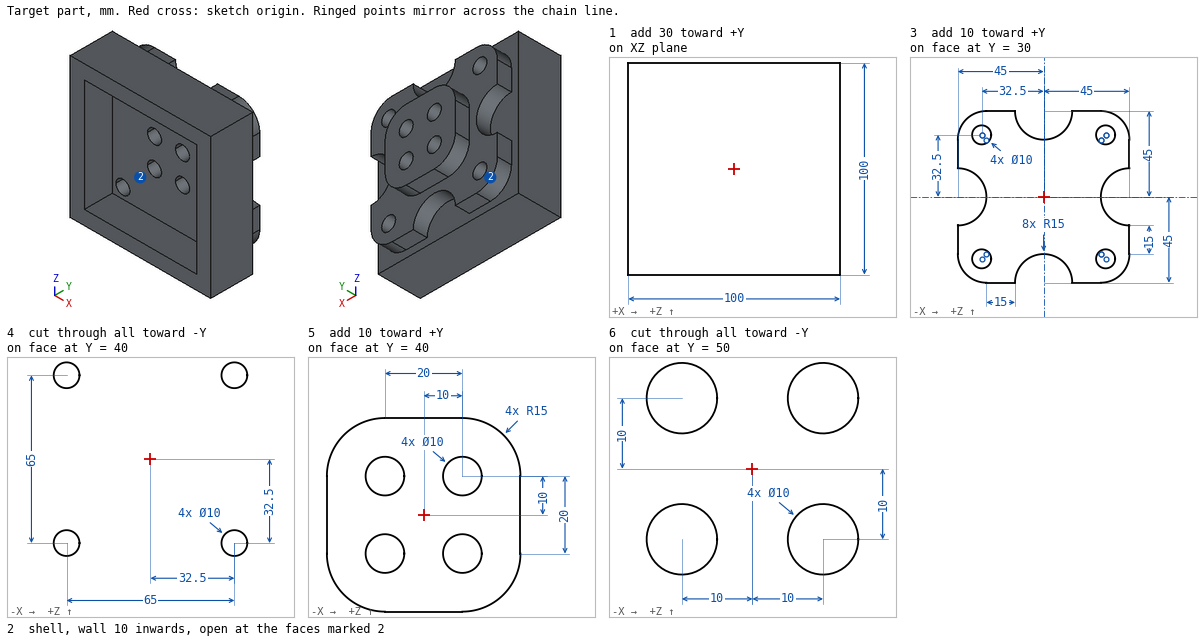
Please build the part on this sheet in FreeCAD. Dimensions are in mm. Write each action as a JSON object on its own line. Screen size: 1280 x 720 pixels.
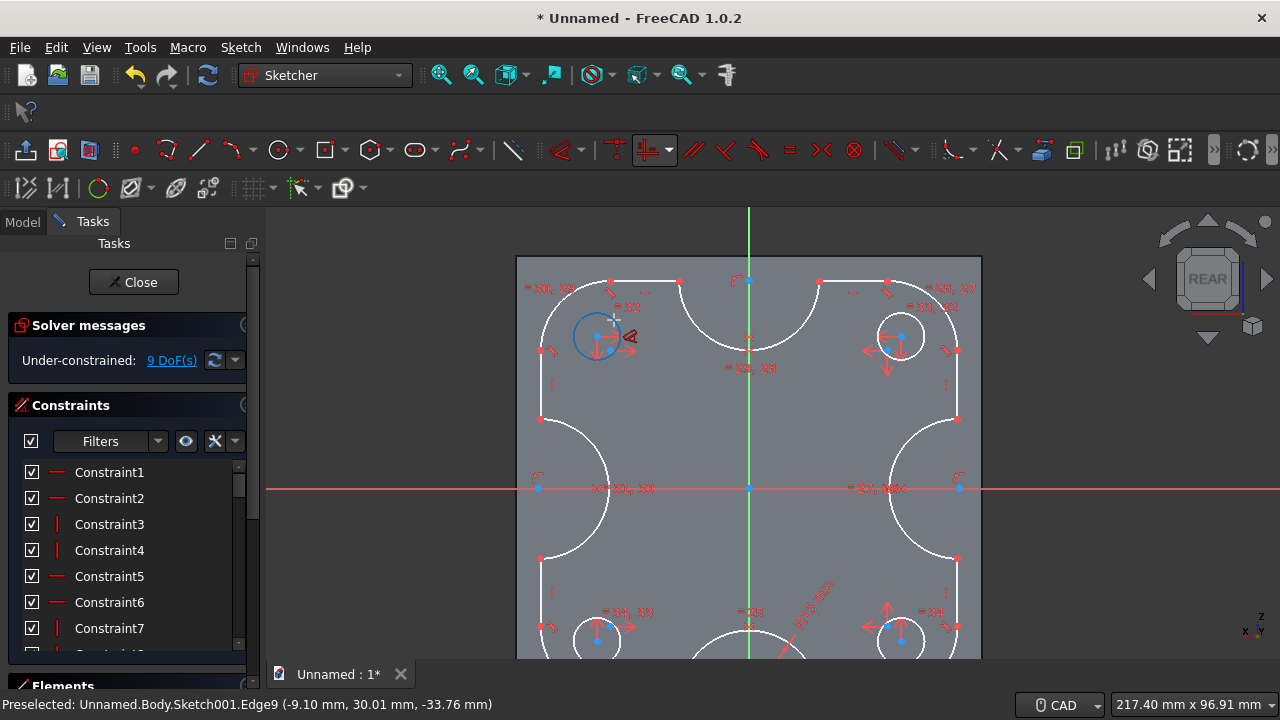
{"action": "left_click", "coordinate": [614, 320]}
{"action": "left_click", "coordinate": [637, 298]}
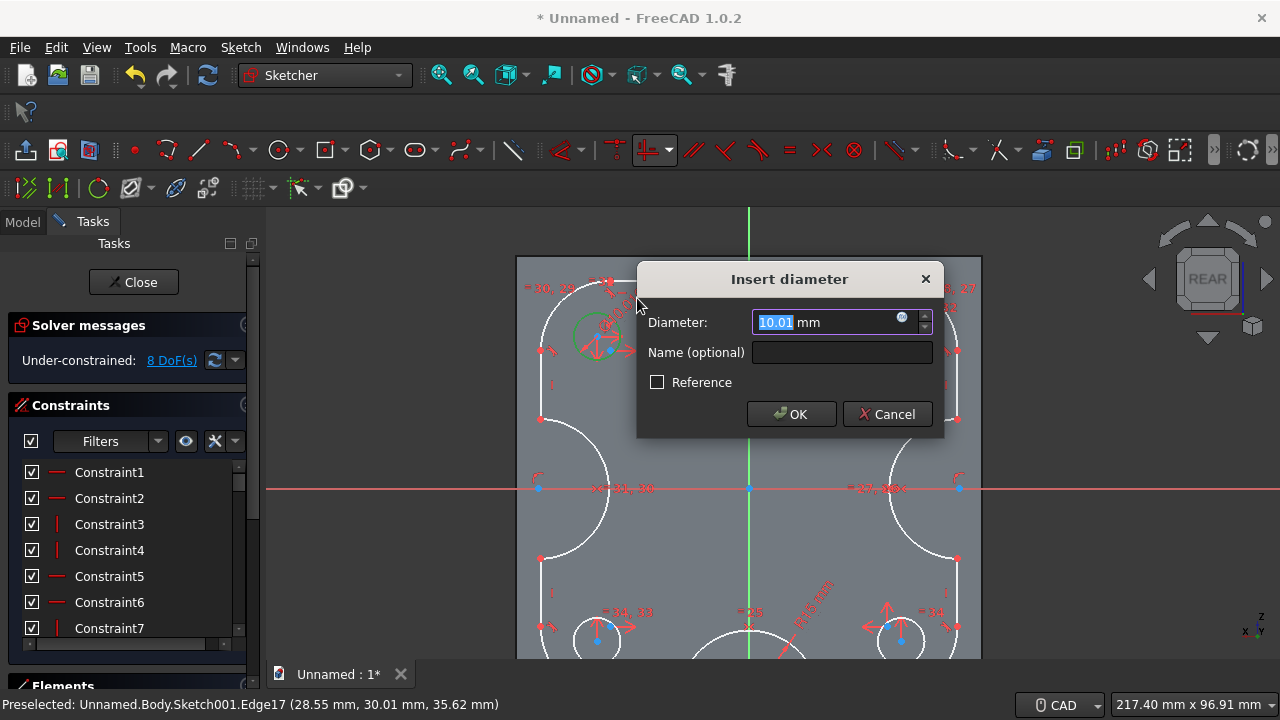
{"action": "type", "text": "10"}
{"action": "key", "text": "Return"}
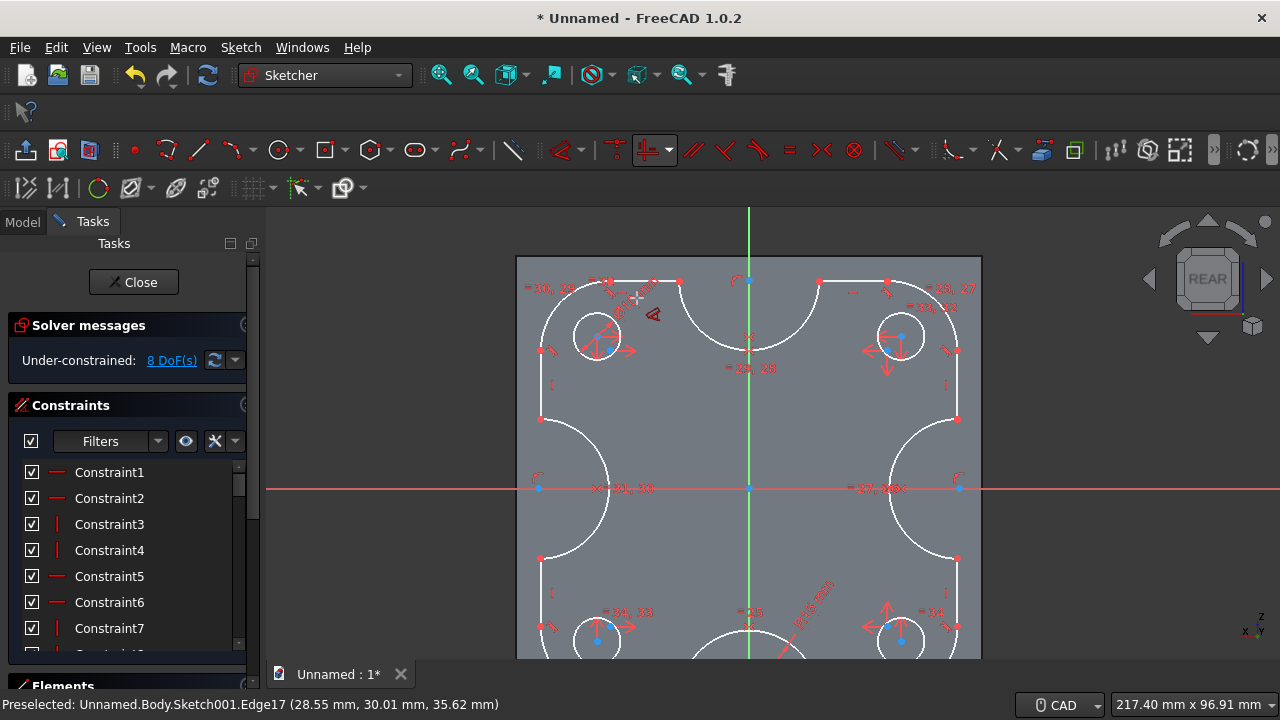
{"action": "scroll", "coordinate": [614, 319], "scroll_direction": "down", "scroll_amount": 2}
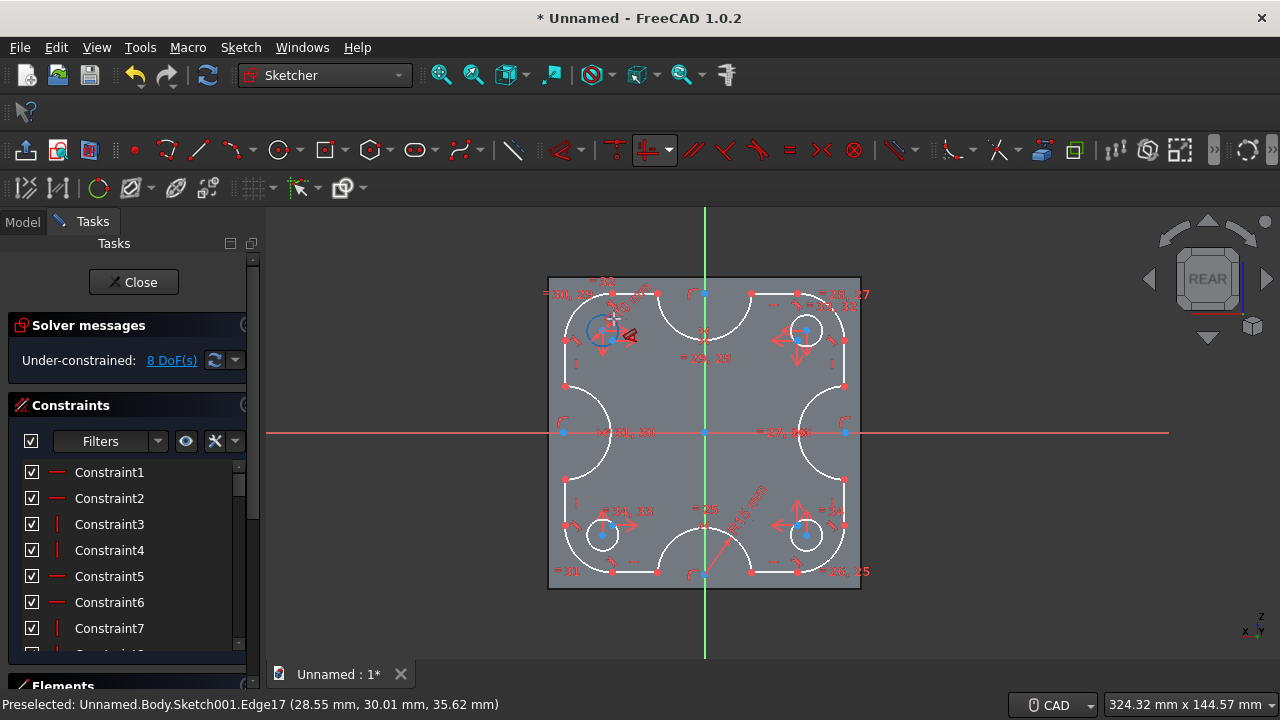
{"action": "left_click", "coordinate": [626, 572]}
{"action": "left_click", "coordinate": [635, 606]}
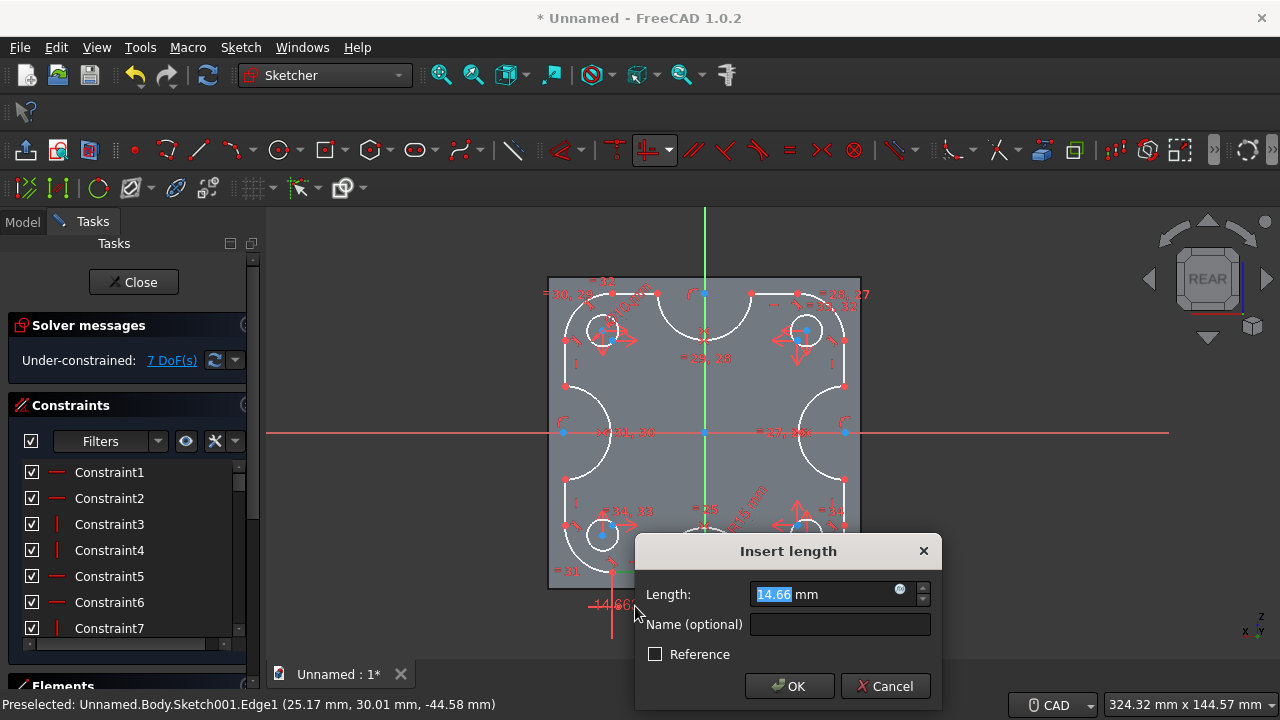
{"action": "type", "text": "15"}
{"action": "key", "text": "Return"}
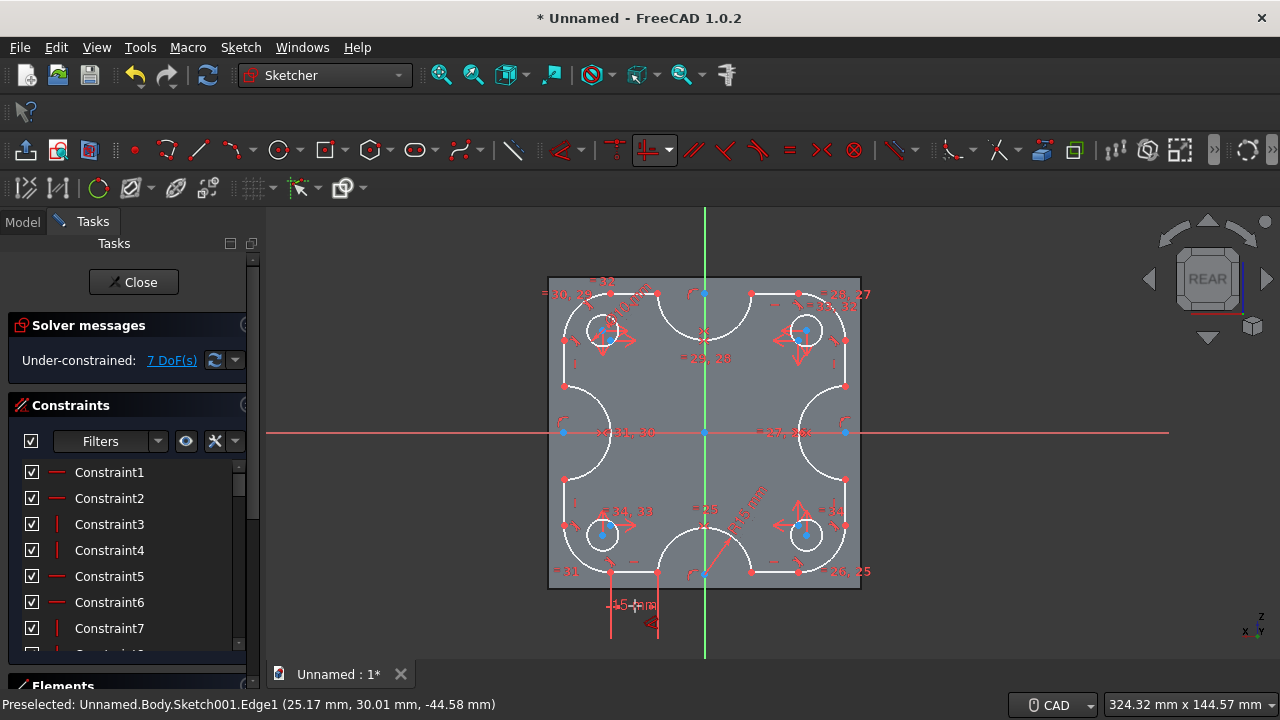
{"action": "left_click", "coordinate": [845, 512]}
{"action": "left_click", "coordinate": [879, 503]}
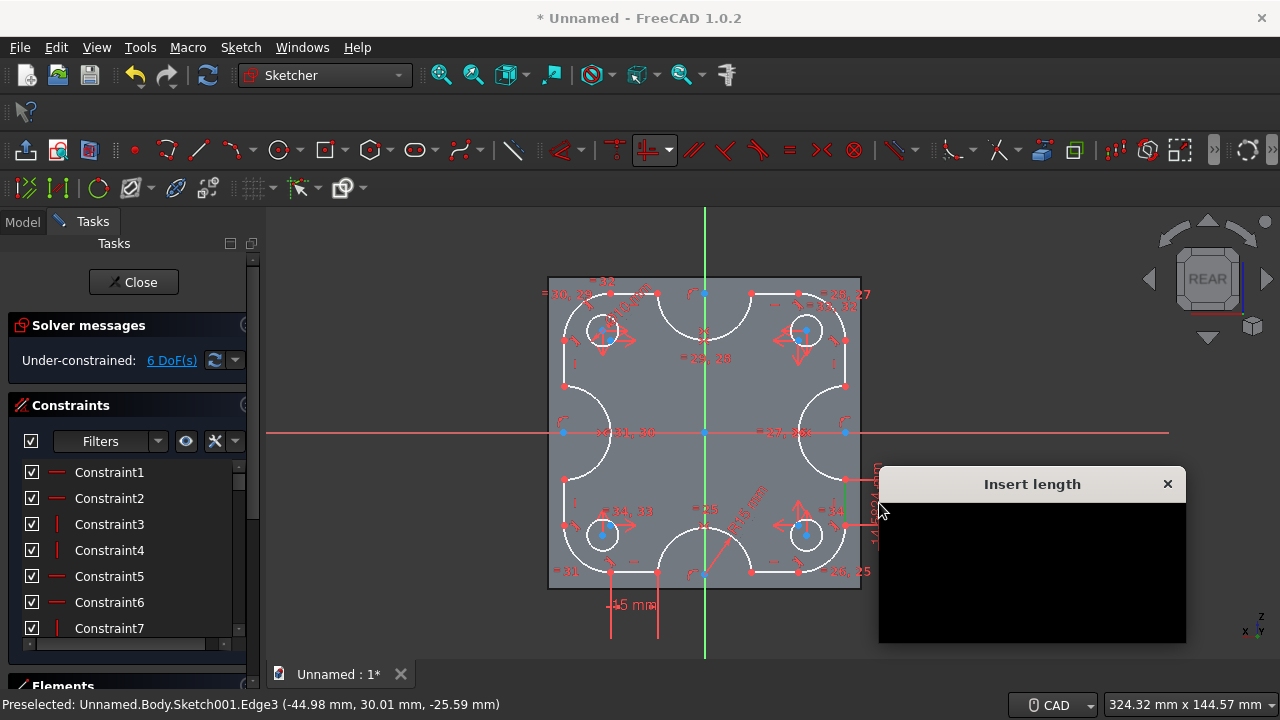
{"action": "type", "text": "15"}
{"action": "key", "text": "Return"}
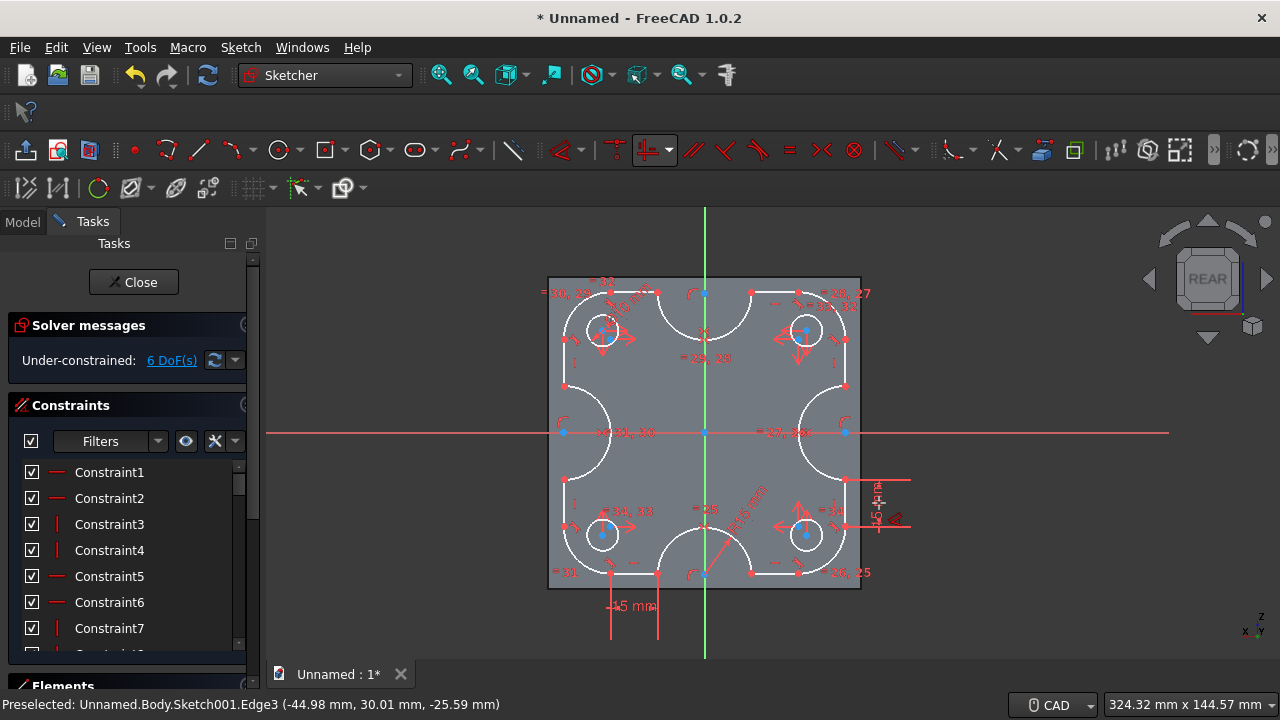
{"action": "left_click", "coordinate": [705, 575]}
{"action": "left_click", "coordinate": [739, 471]}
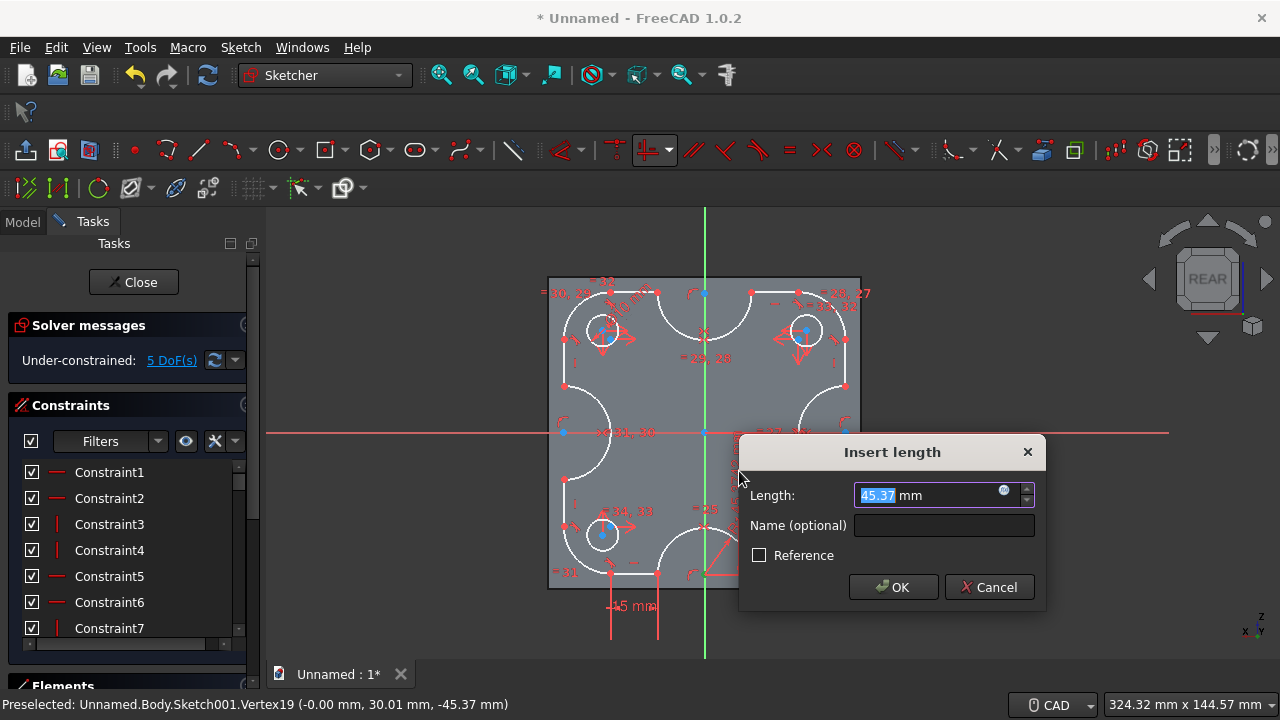
{"action": "type", "text": "45"}
{"action": "key", "text": "Return"}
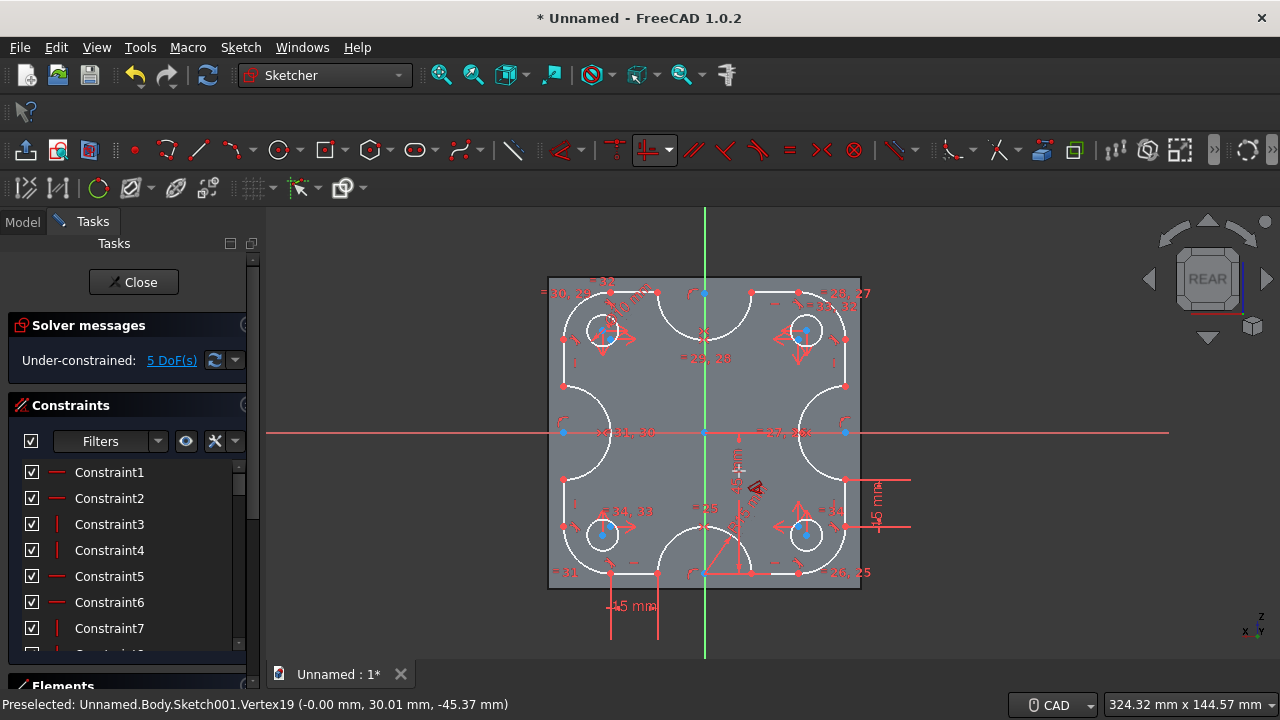
{"action": "left_click", "coordinate": [846, 433]}
{"action": "left_click", "coordinate": [775, 399]}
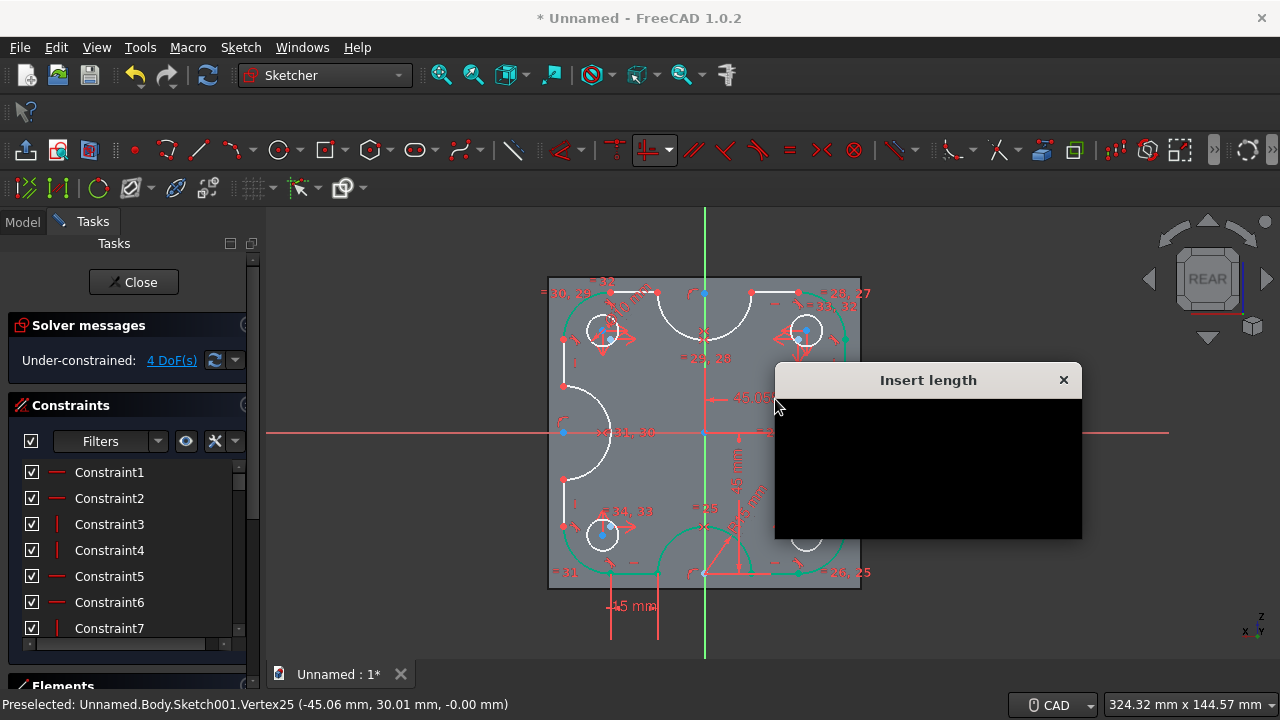
{"action": "type", "text": "45"}
{"action": "key", "text": "Return"}